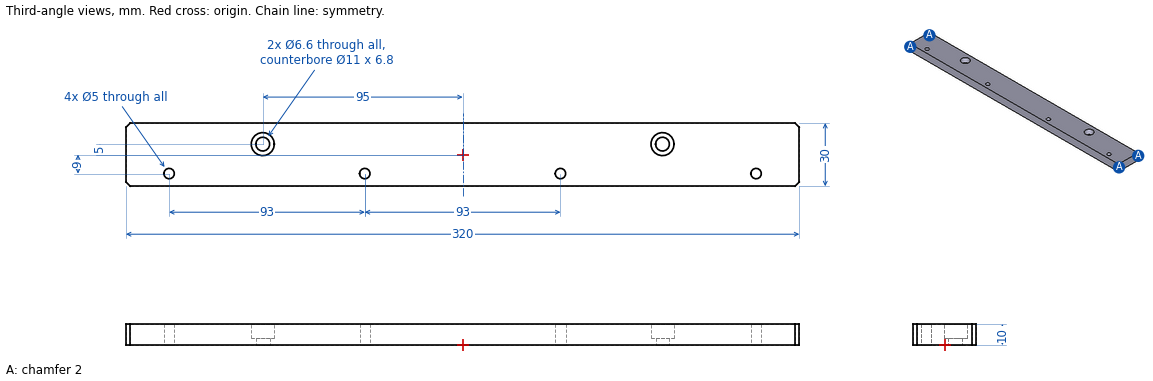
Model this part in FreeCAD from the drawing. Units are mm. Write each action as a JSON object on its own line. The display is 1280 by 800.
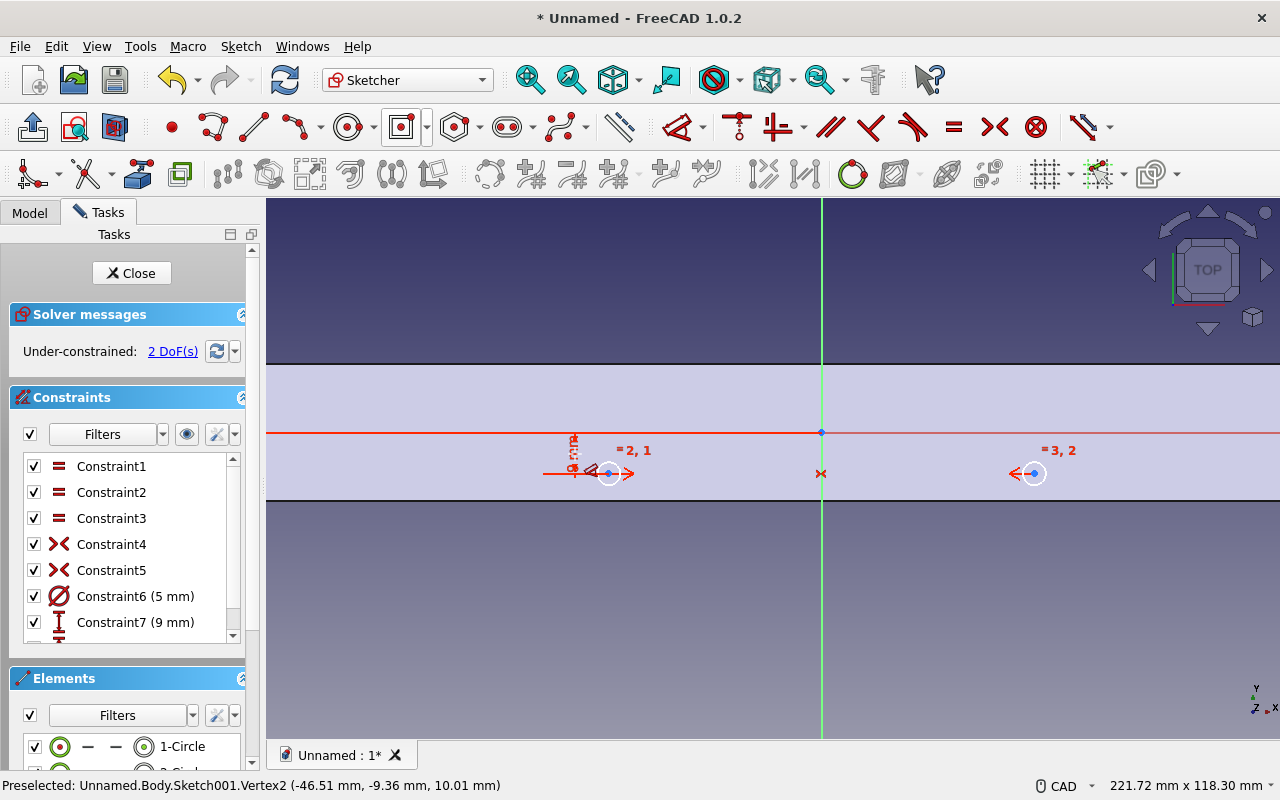
{"action": "scroll", "coordinate": [609, 476], "scroll_direction": "down", "scroll_amount": 4}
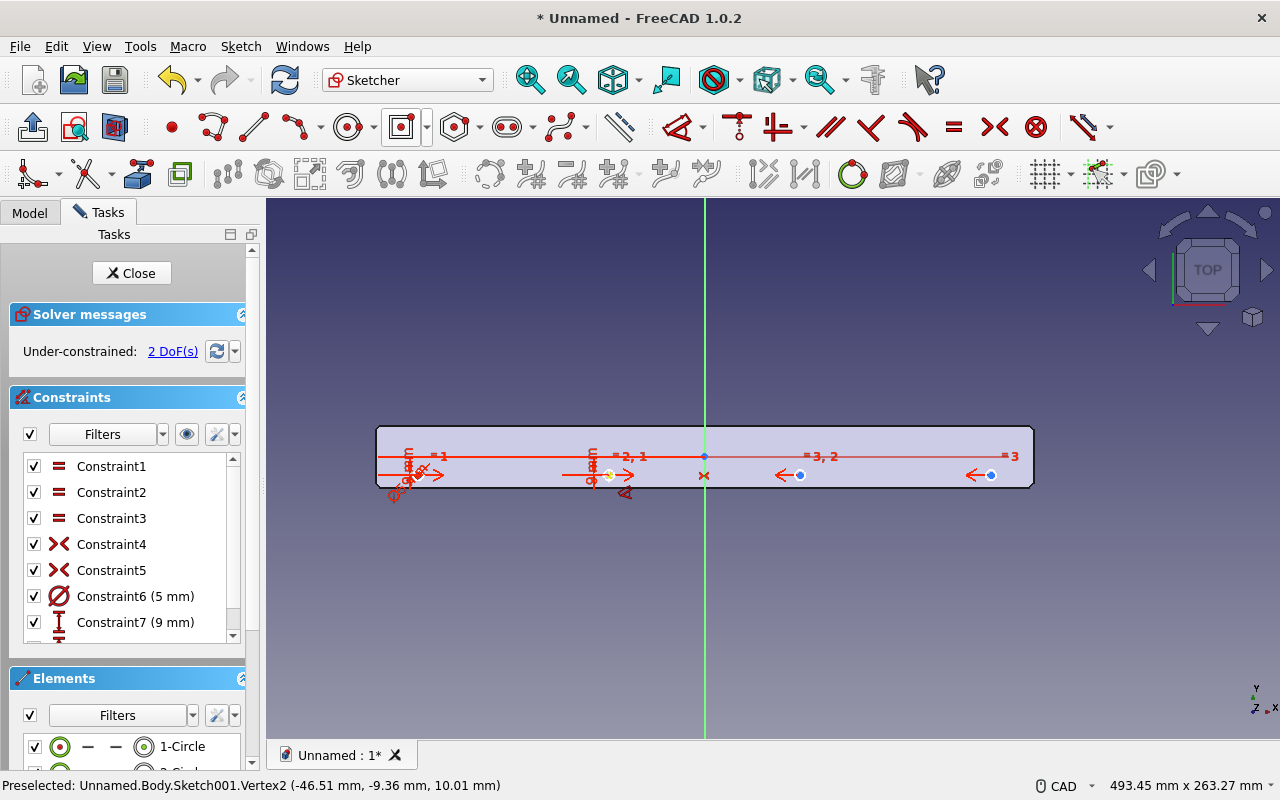
{"action": "left_click", "coordinate": [418, 475]}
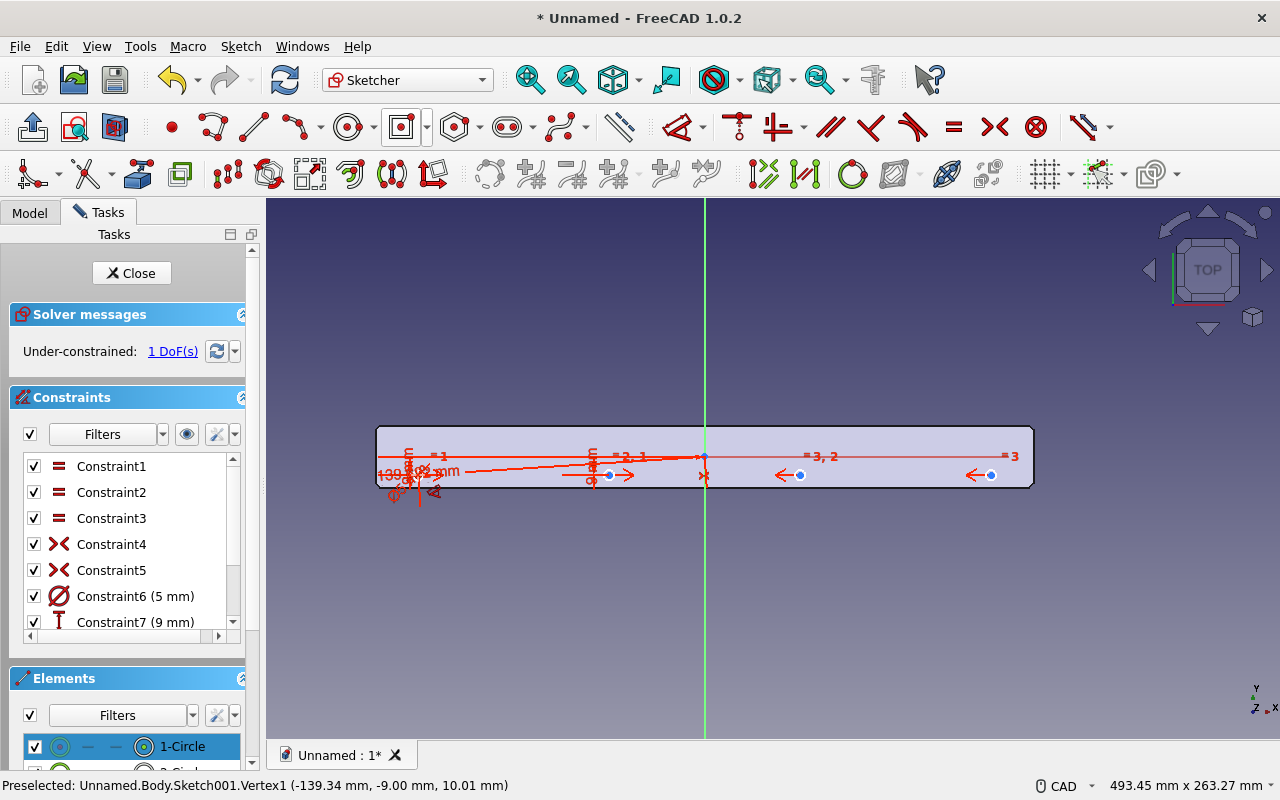
{"action": "left_click", "coordinate": [609, 475]}
{"action": "left_click", "coordinate": [514, 509]}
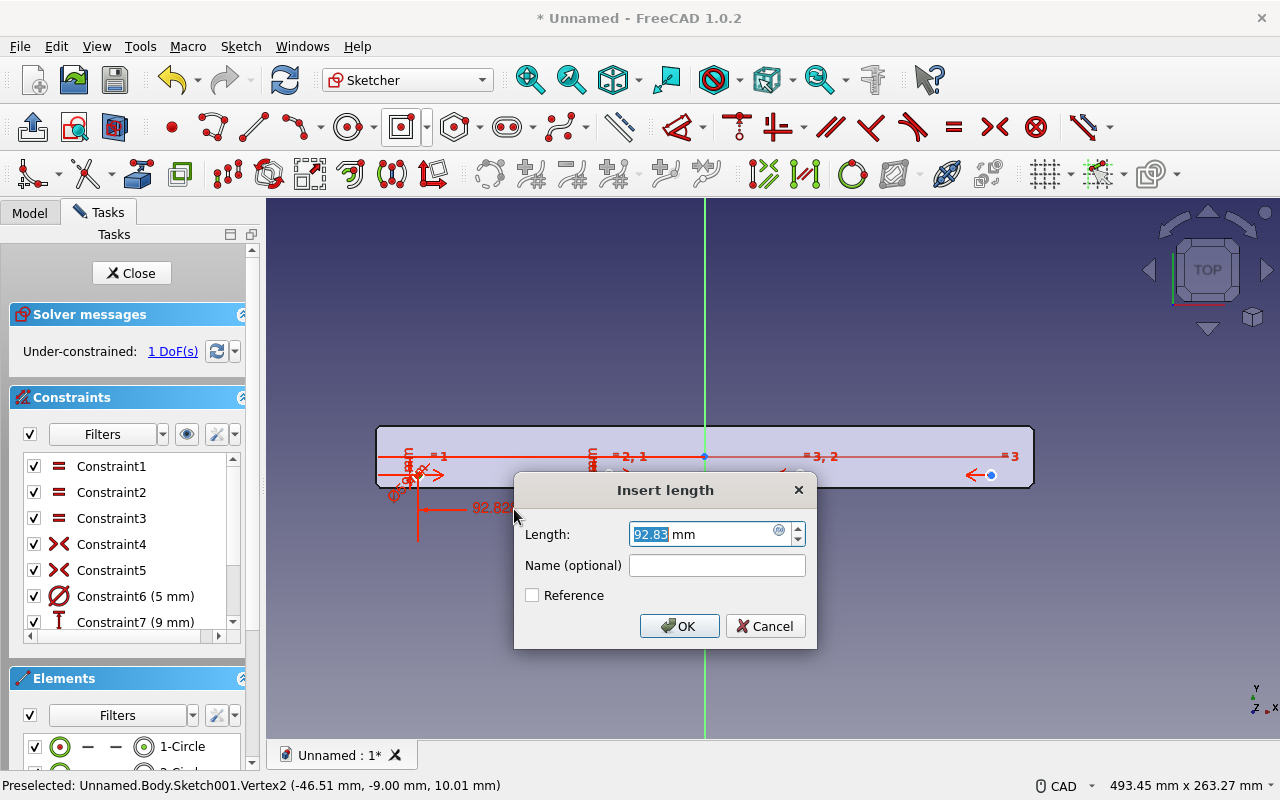
{"action": "type", "text": "93"}
{"action": "key", "text": "Return"}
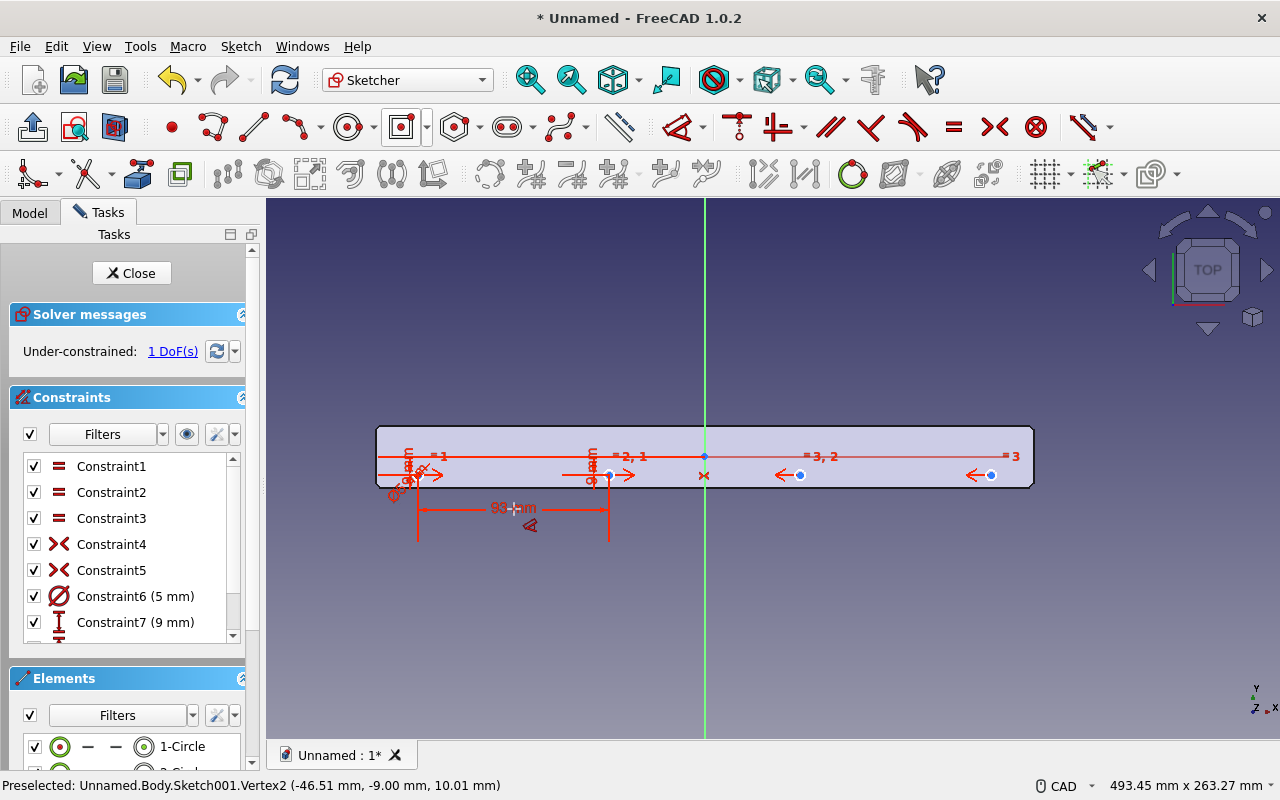
{"action": "left_click", "coordinate": [609, 475]}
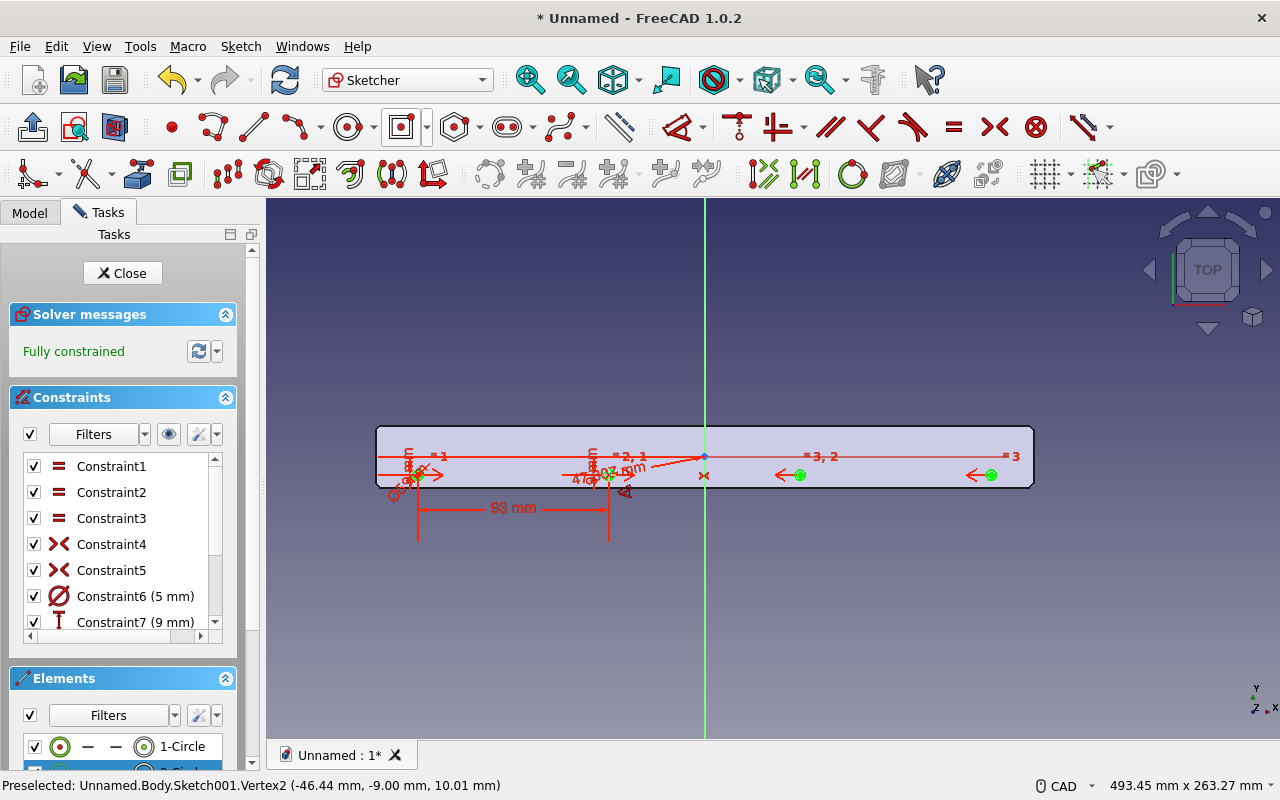
{"action": "left_click", "coordinate": [800, 475]}
{"action": "left_click", "coordinate": [661, 509]}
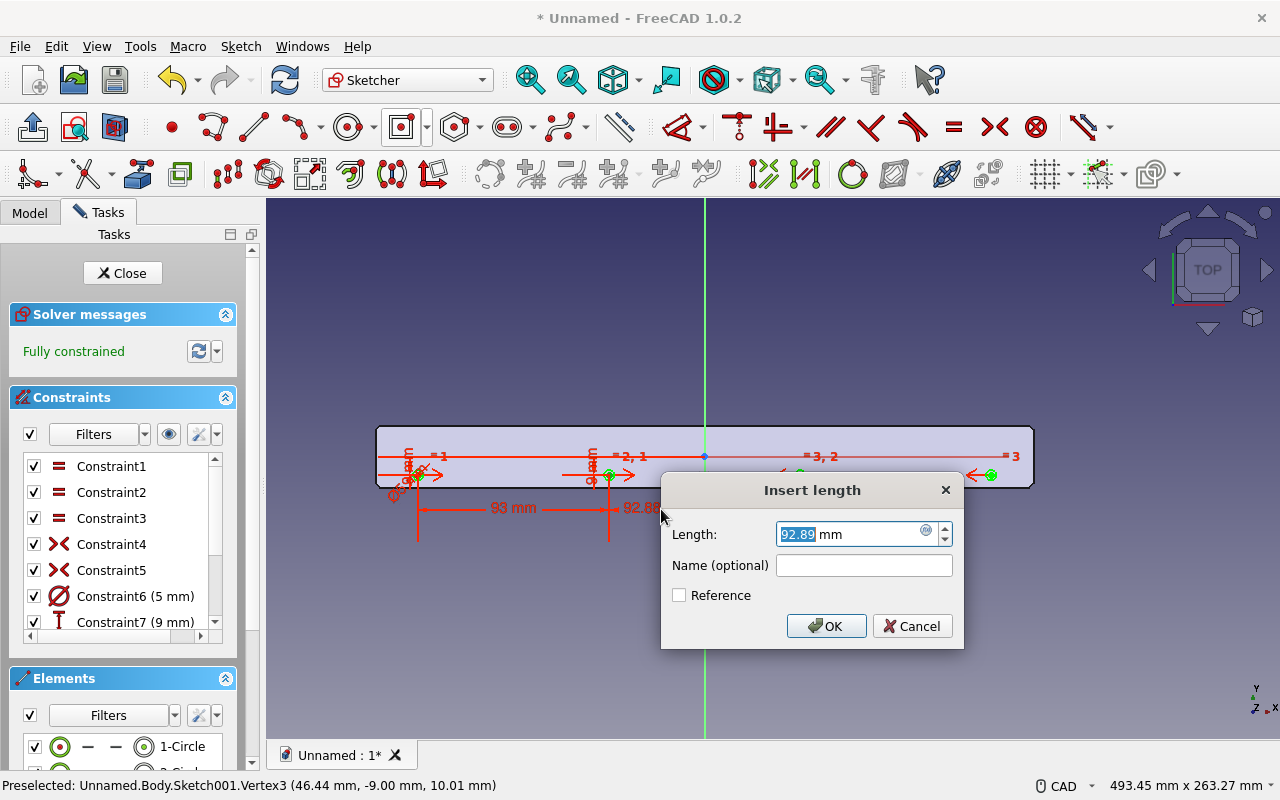
{"action": "type", "text": "93"}
{"action": "key", "text": "Return"}
{"action": "key", "text": "Escape"}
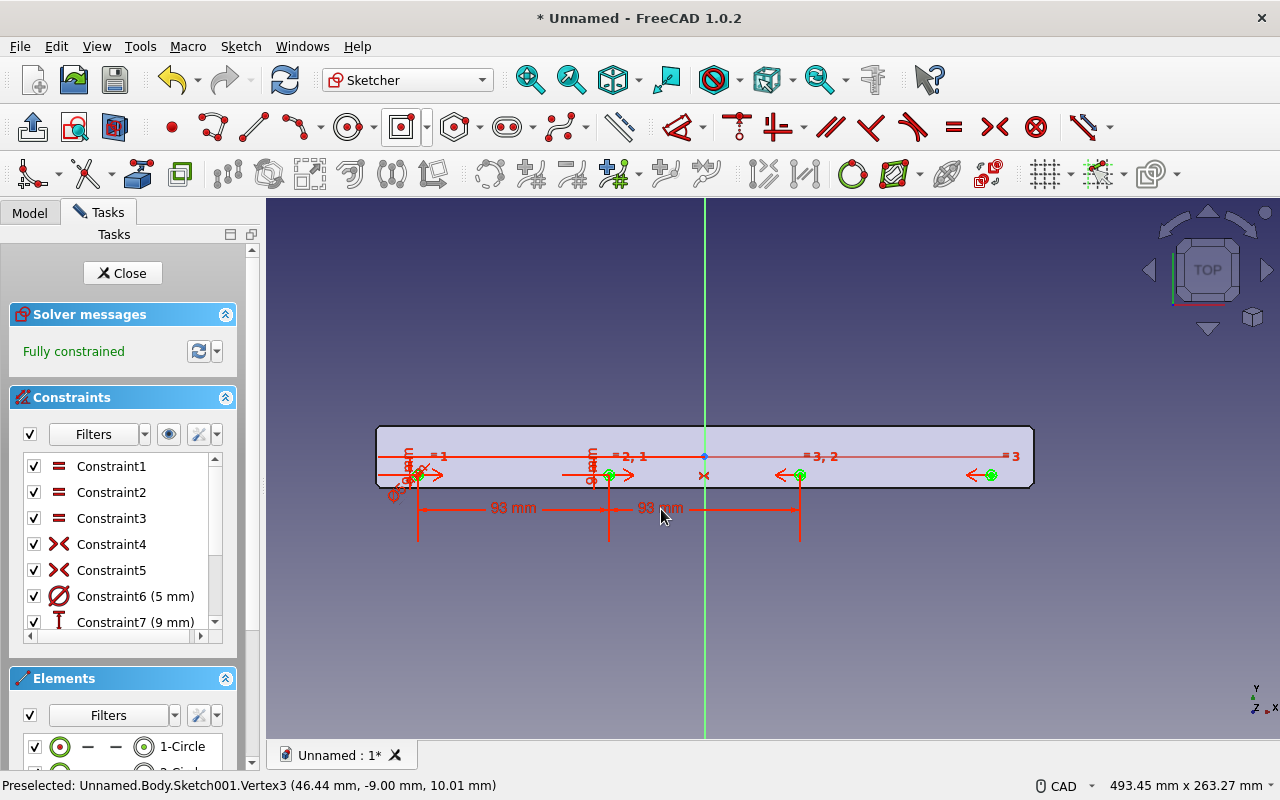
{"action": "left_click", "coordinate": [123, 273]}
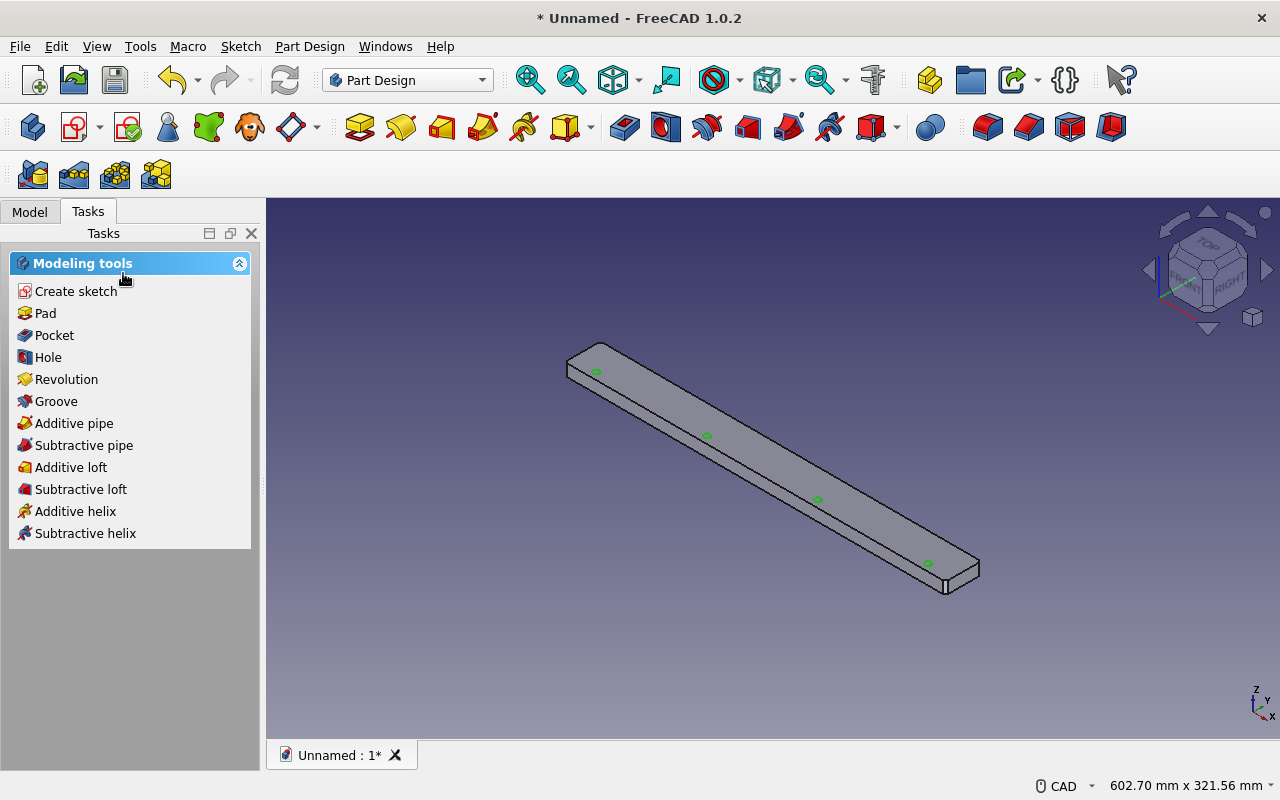
{"action": "left_click", "coordinate": [666, 128]}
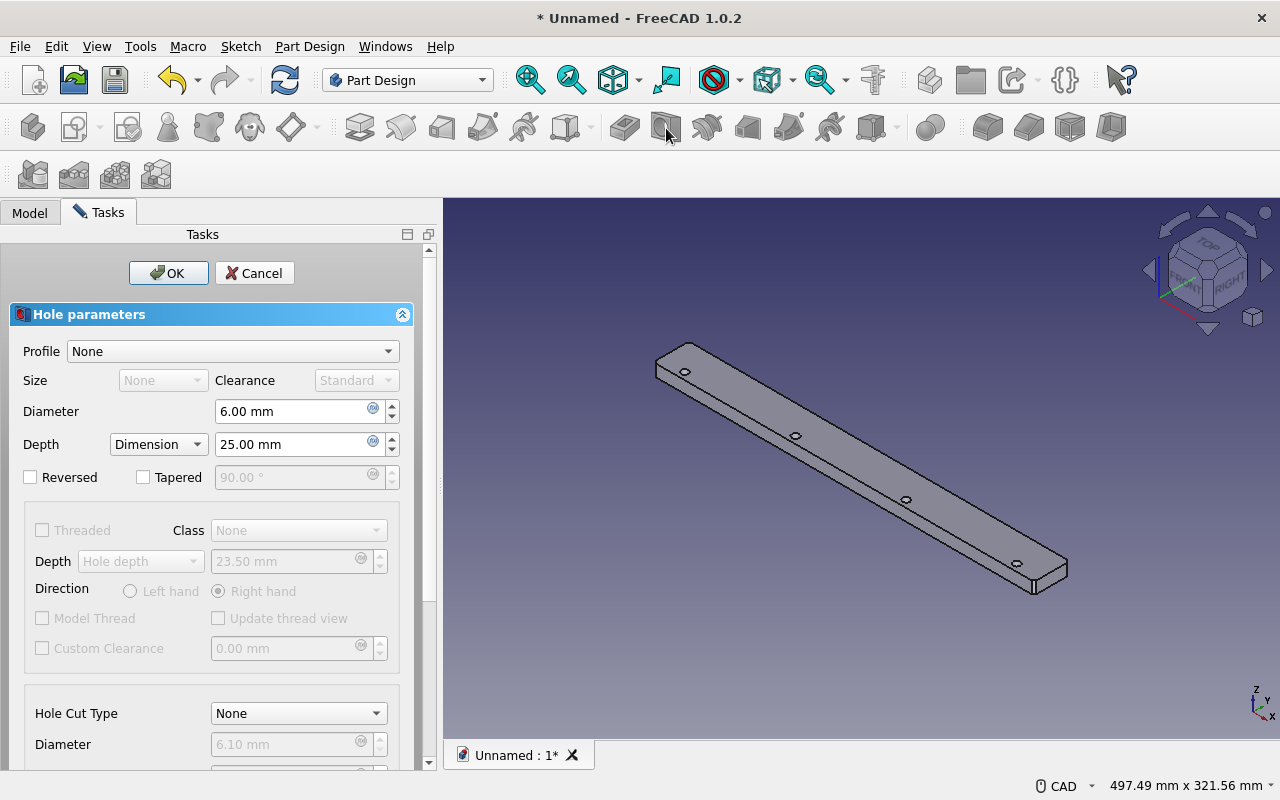
{"action": "triple_click", "coordinate": [300, 412]}